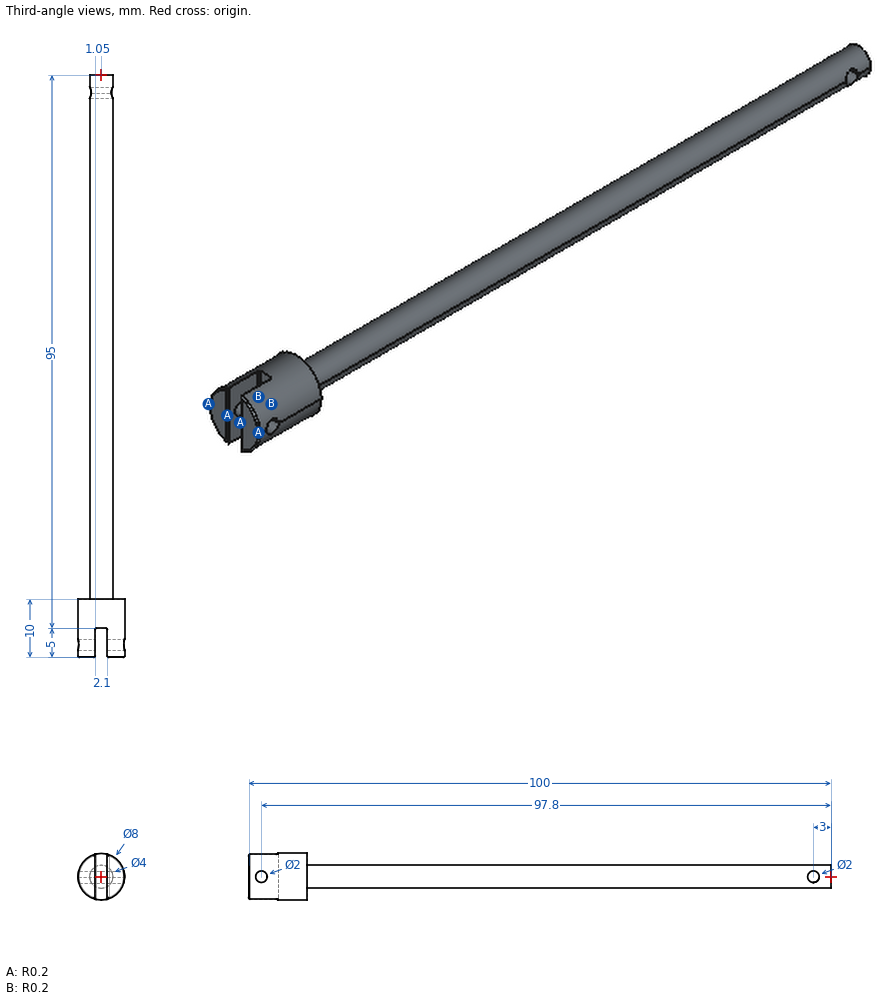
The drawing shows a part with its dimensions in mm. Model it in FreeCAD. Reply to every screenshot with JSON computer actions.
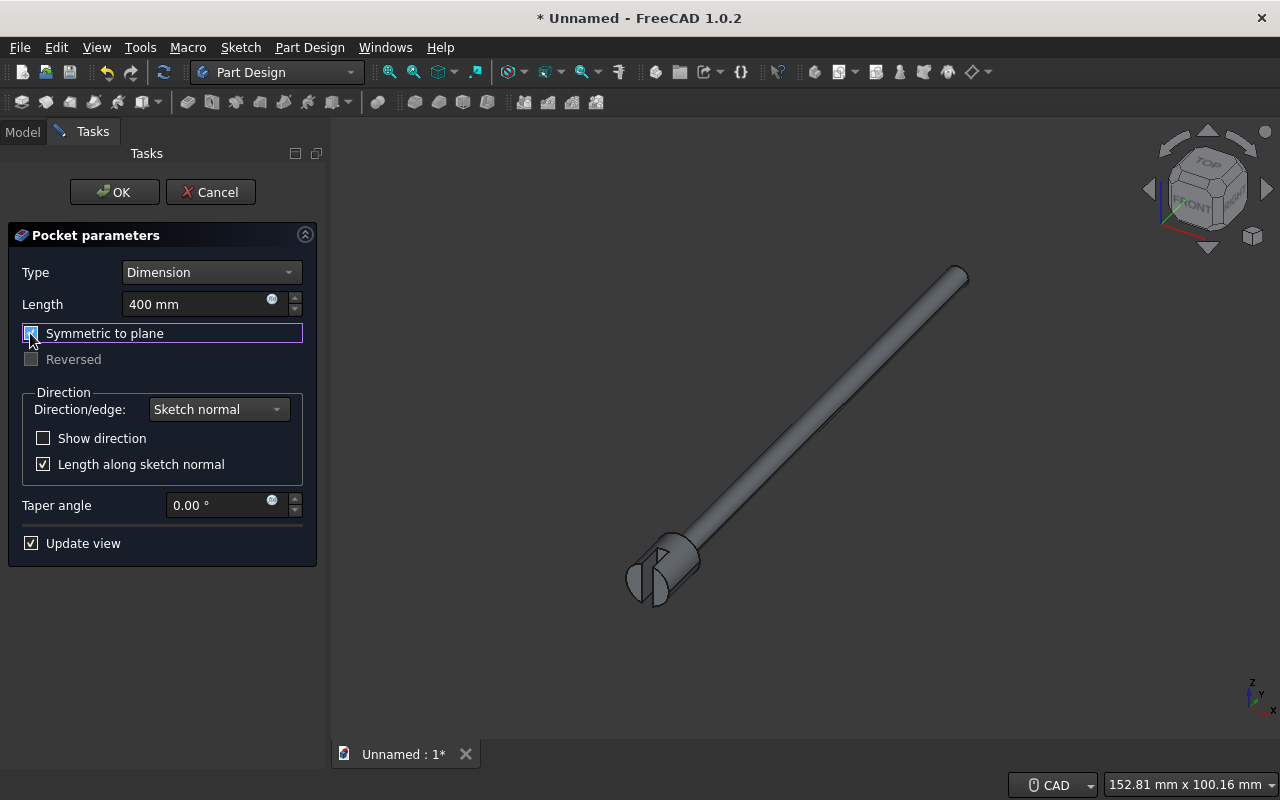
{"action": "left_click", "coordinate": [115, 192]}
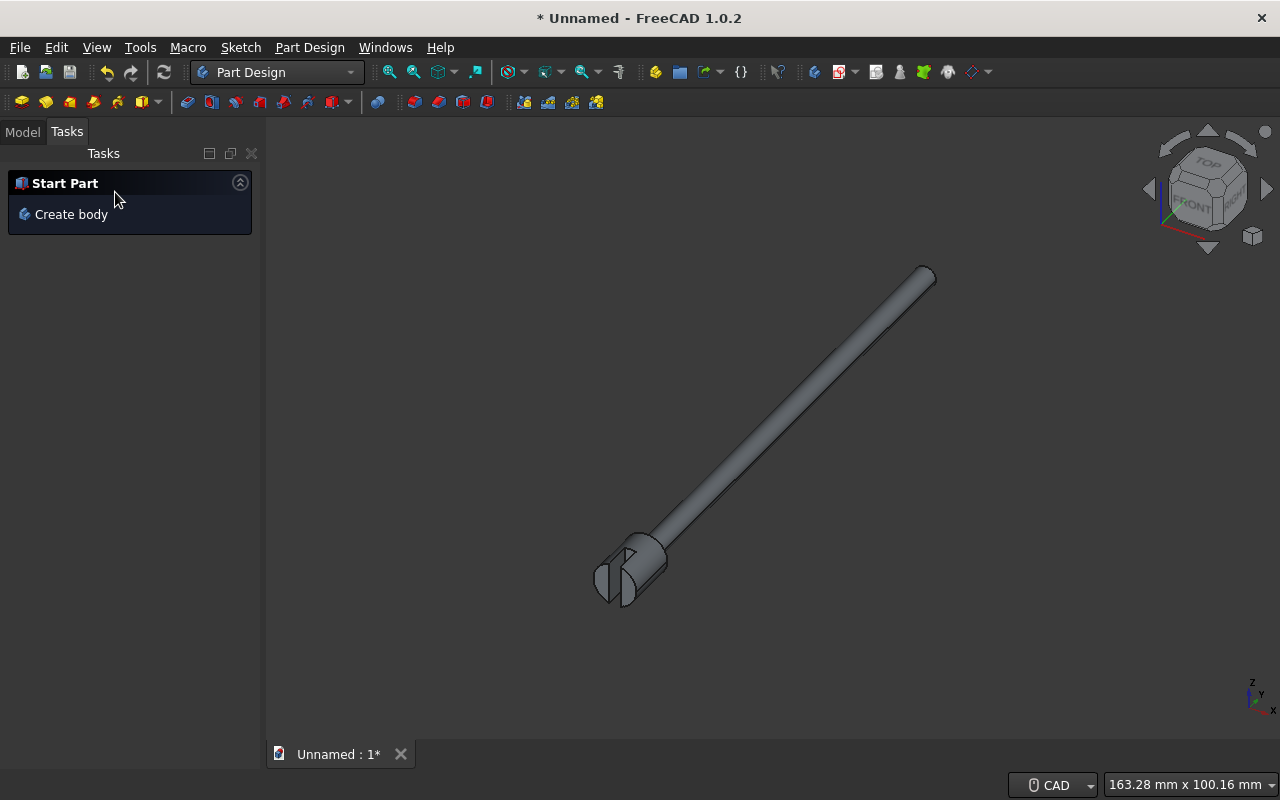
{"action": "left_click", "coordinate": [23, 131]}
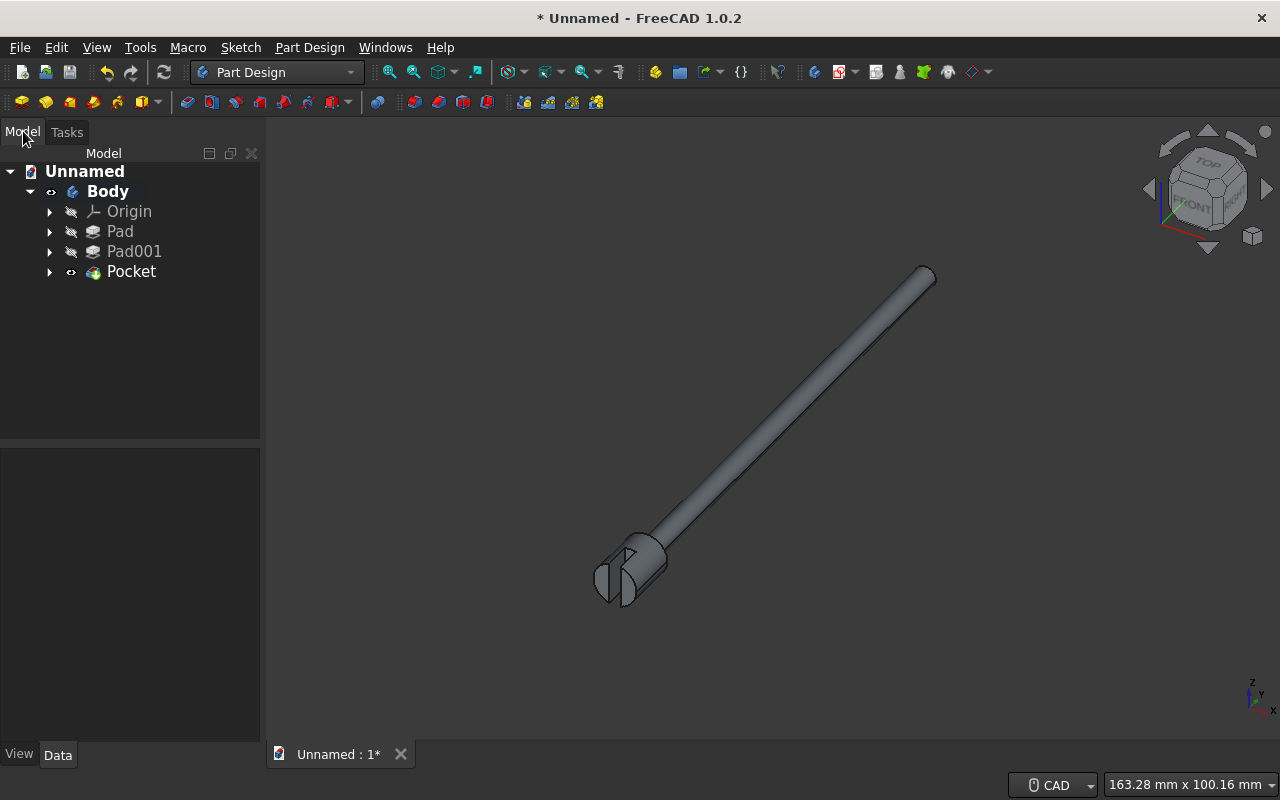
{"action": "left_click", "coordinate": [50, 212]}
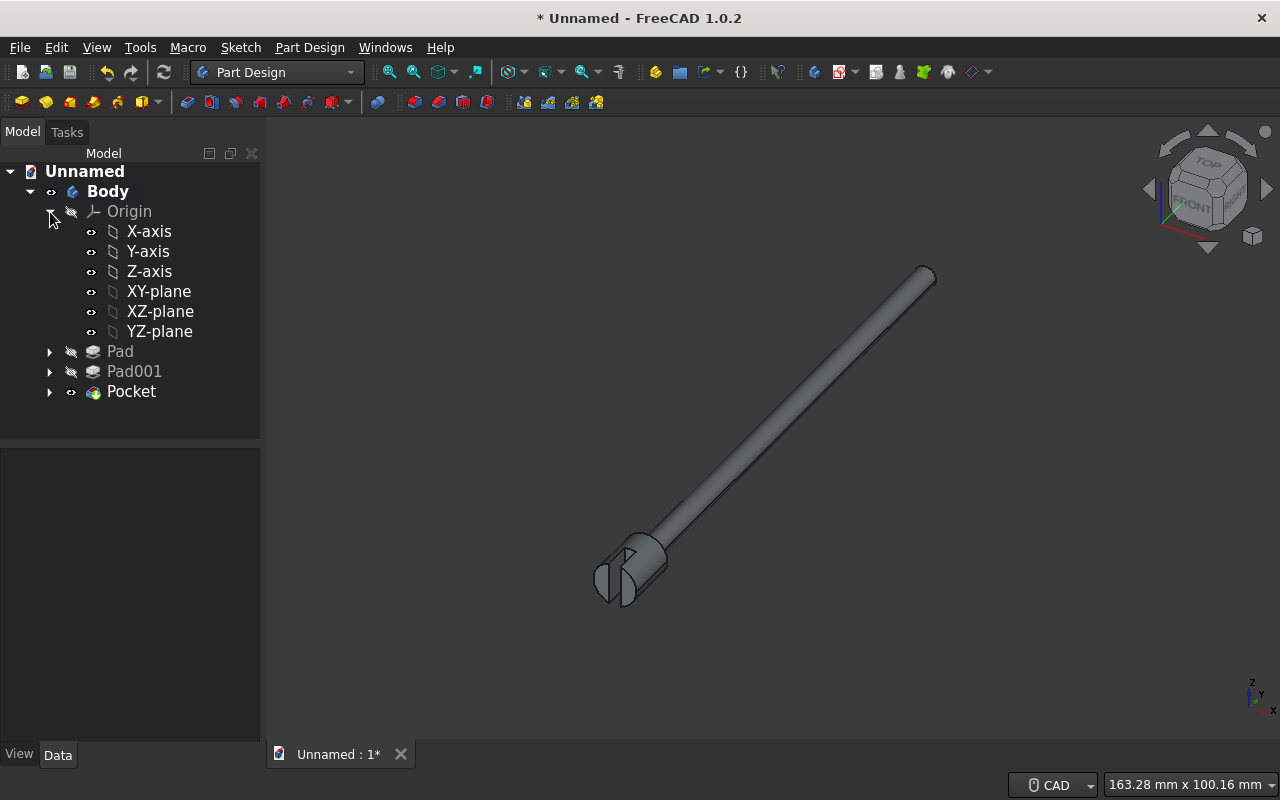
{"action": "left_click", "coordinate": [136, 332]}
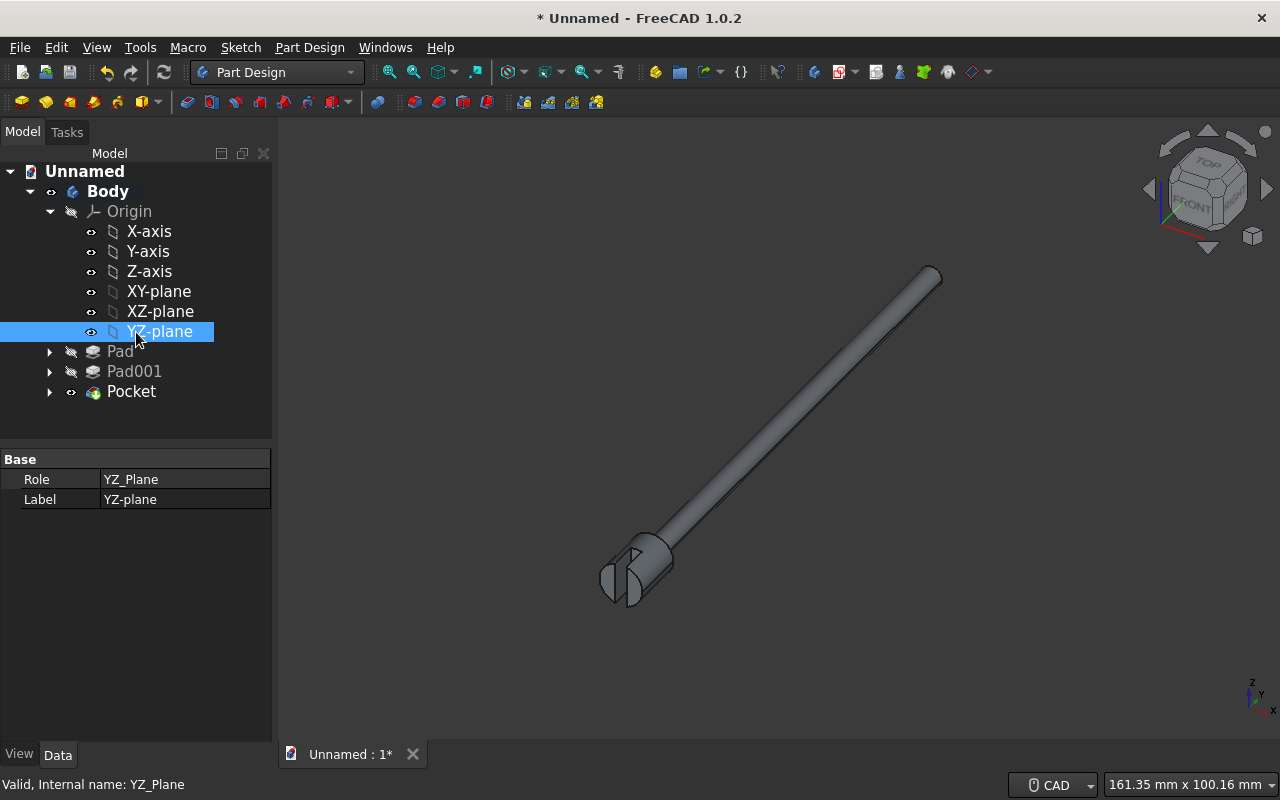
{"action": "left_click", "coordinate": [972, 72]}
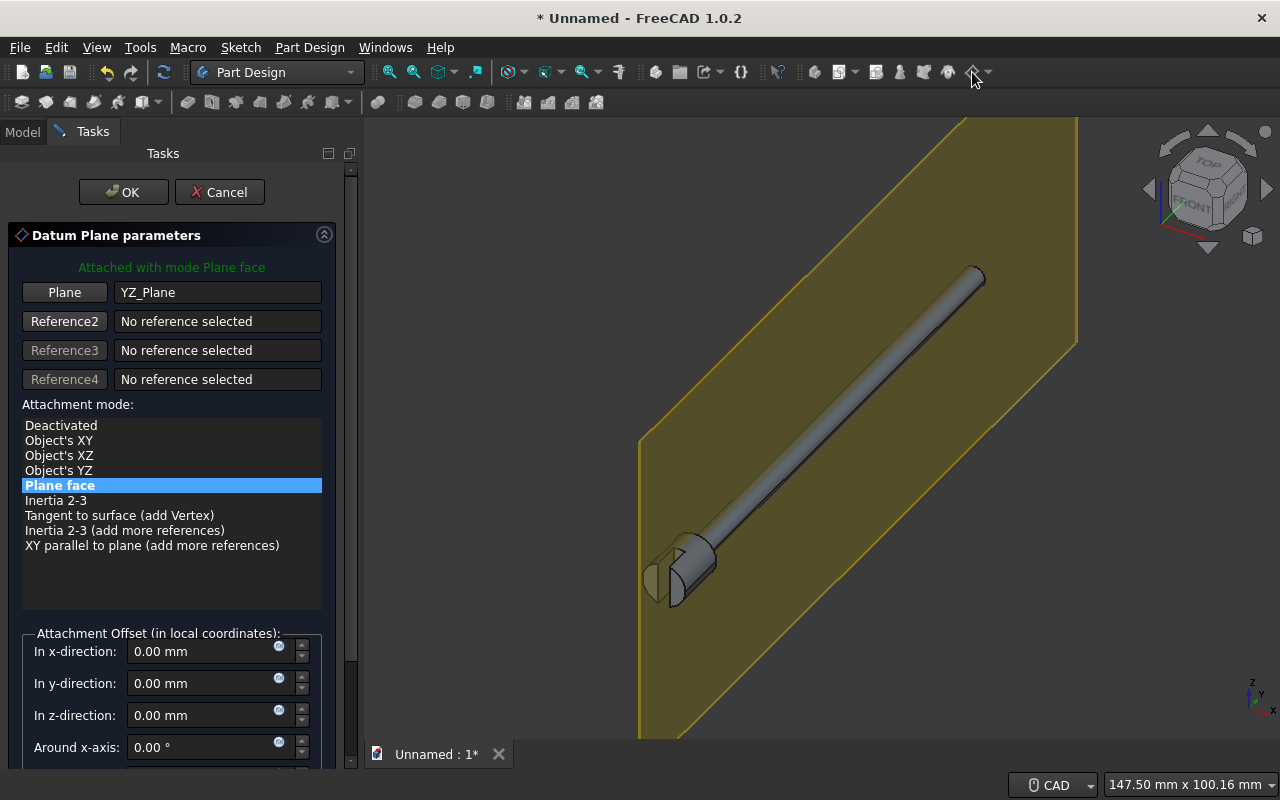
{"action": "triple_click", "coordinate": [210, 715]}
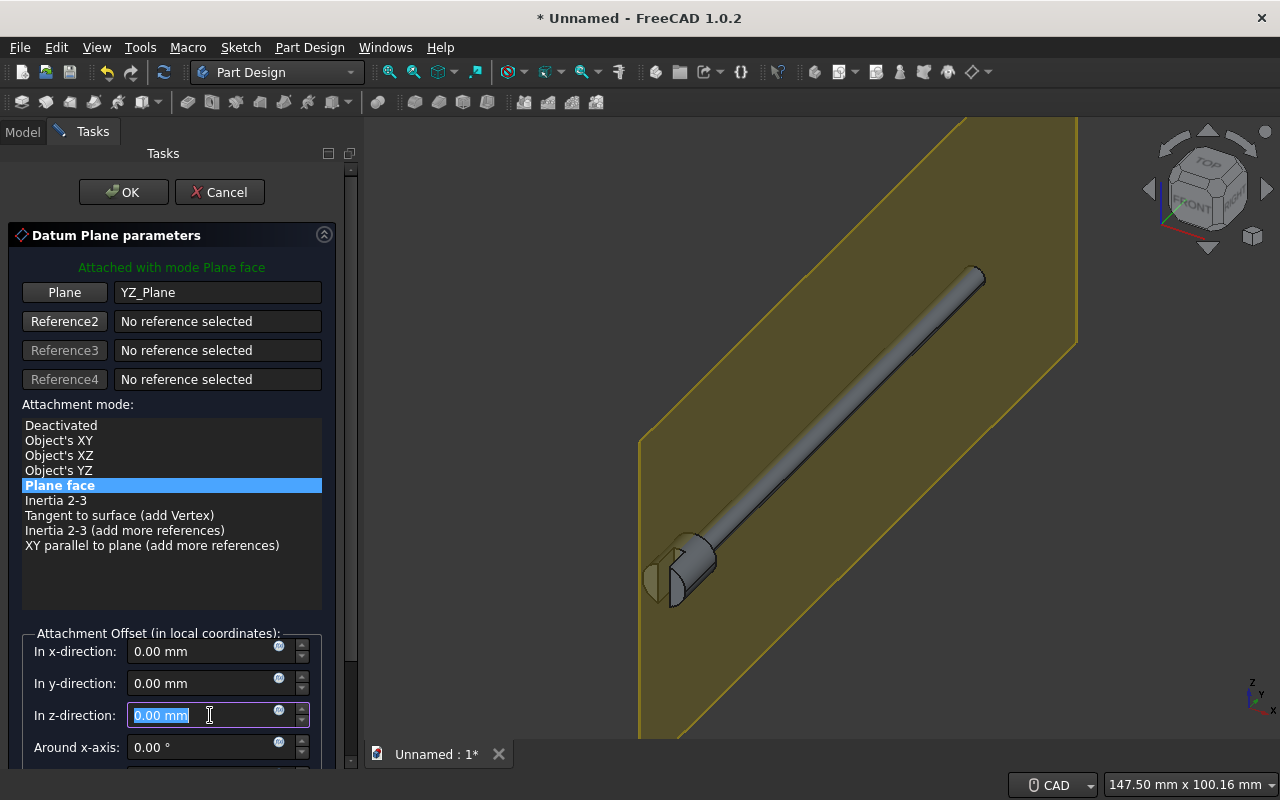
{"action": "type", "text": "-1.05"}
{"action": "key", "text": "Tab"}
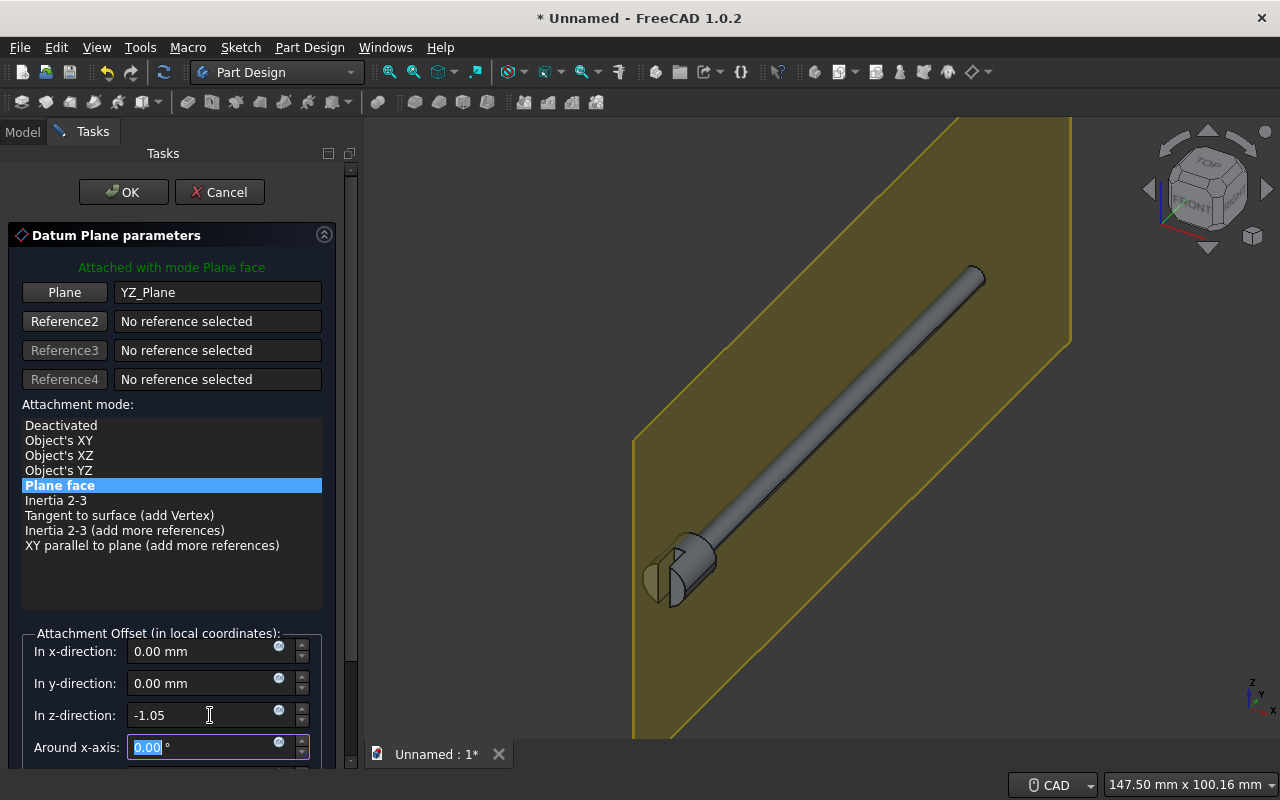
{"action": "left_click", "coordinate": [124, 192]}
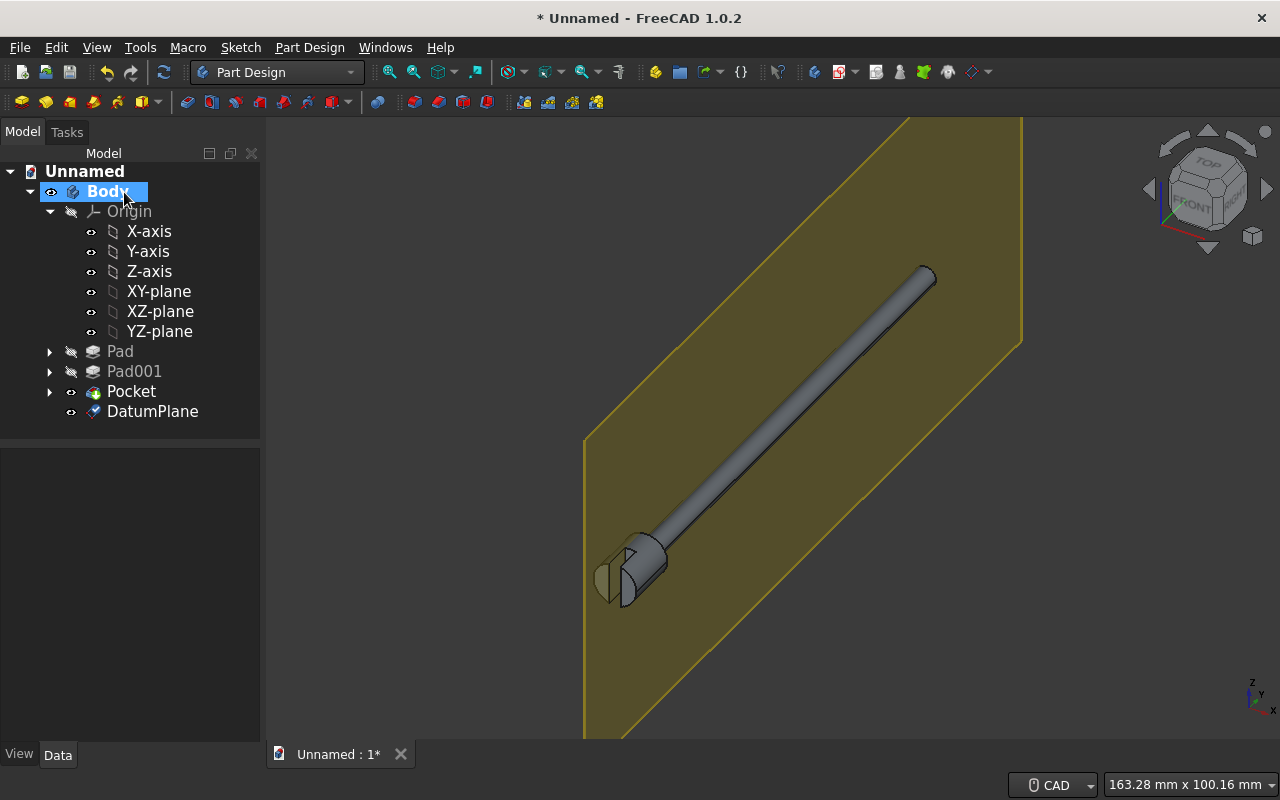
{"action": "left_click", "coordinate": [116, 412]}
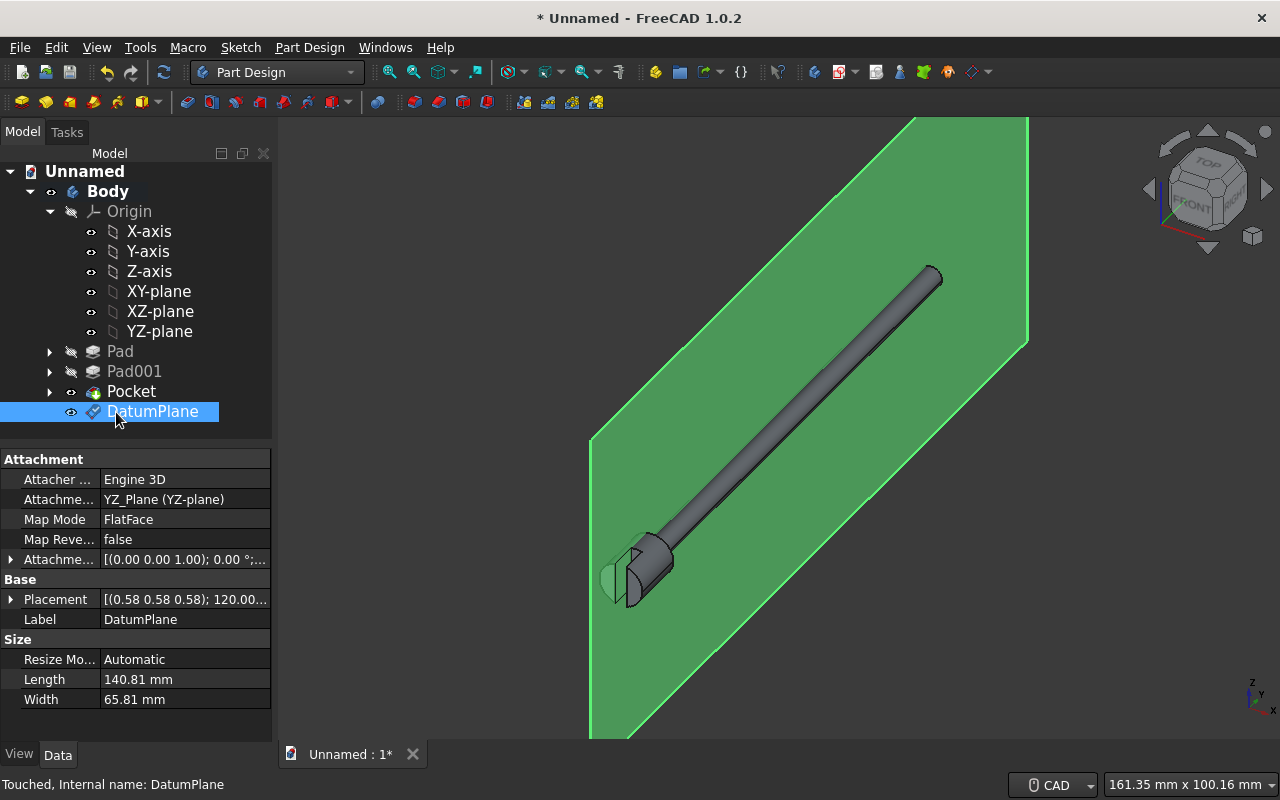
{"action": "left_click", "coordinate": [840, 72]}